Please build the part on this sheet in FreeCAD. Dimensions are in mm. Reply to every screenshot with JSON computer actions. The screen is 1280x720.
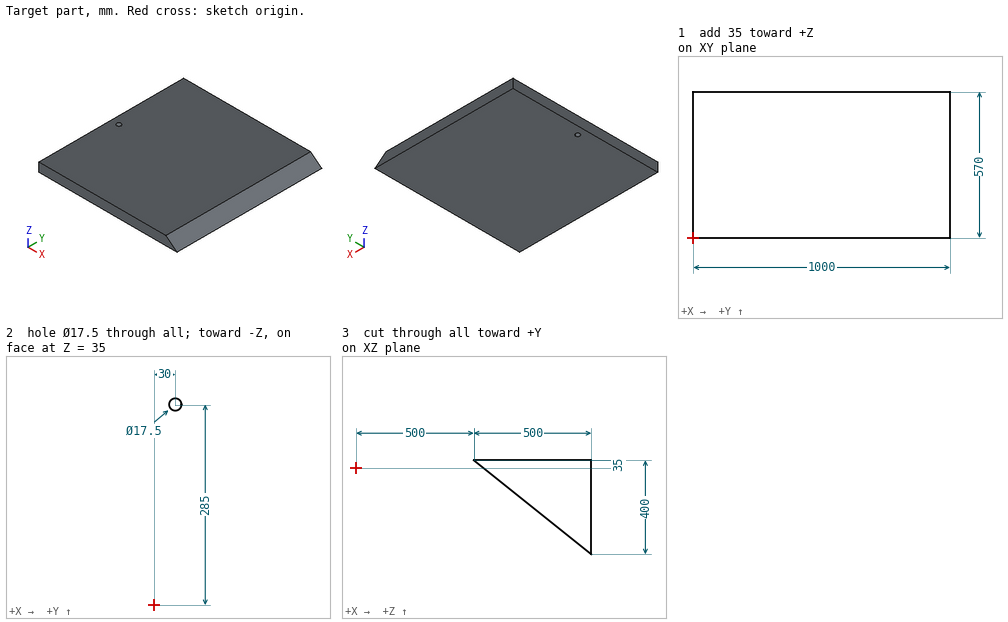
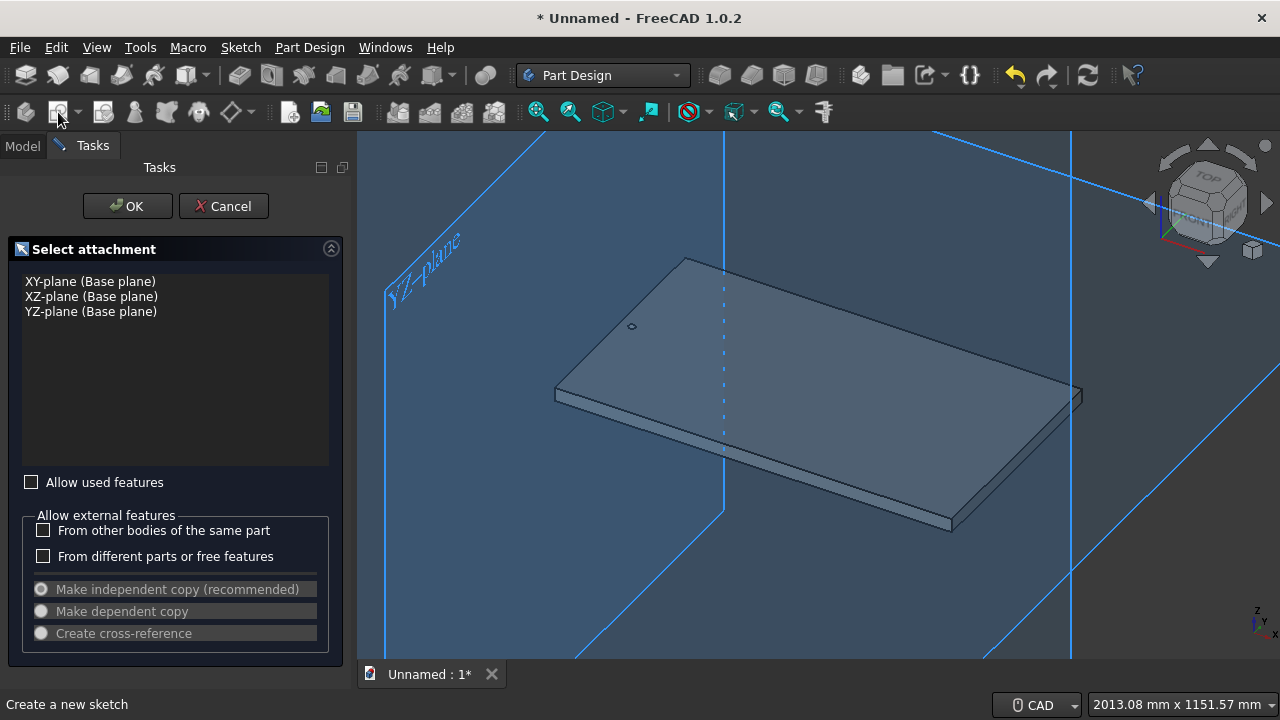
{"action": "left_click", "coordinate": [82, 296]}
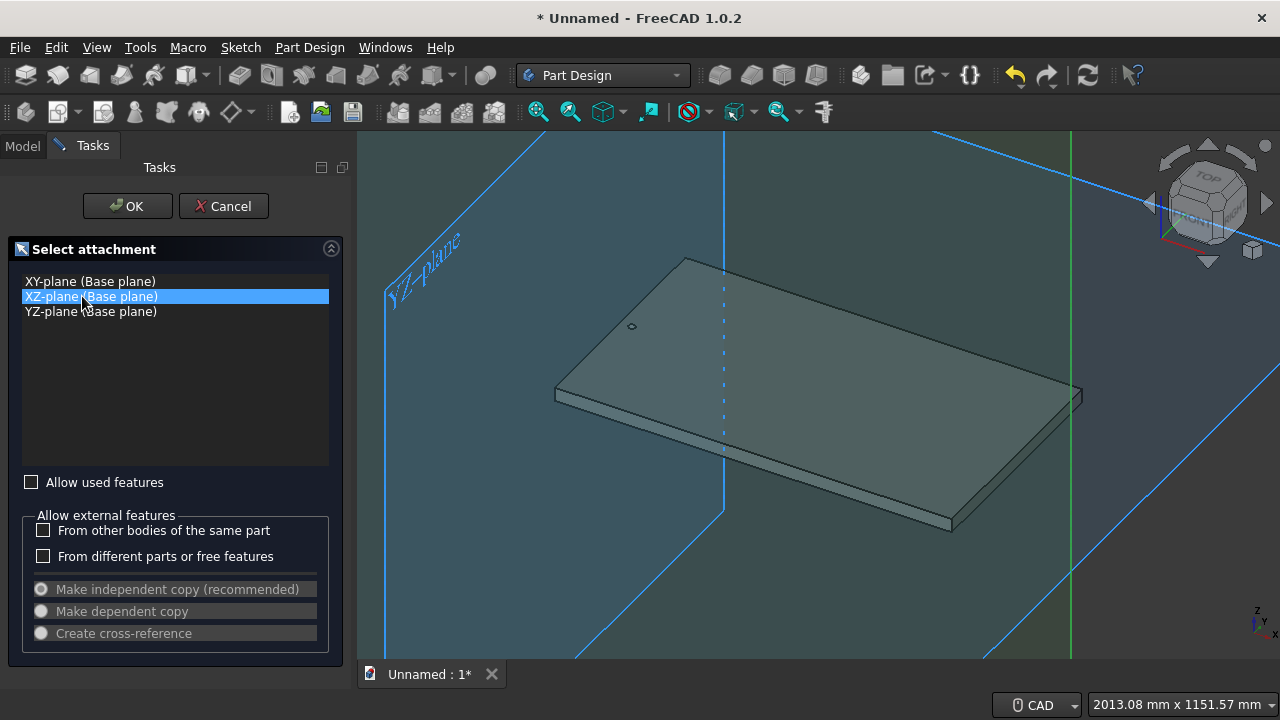
{"action": "left_click", "coordinate": [128, 206]}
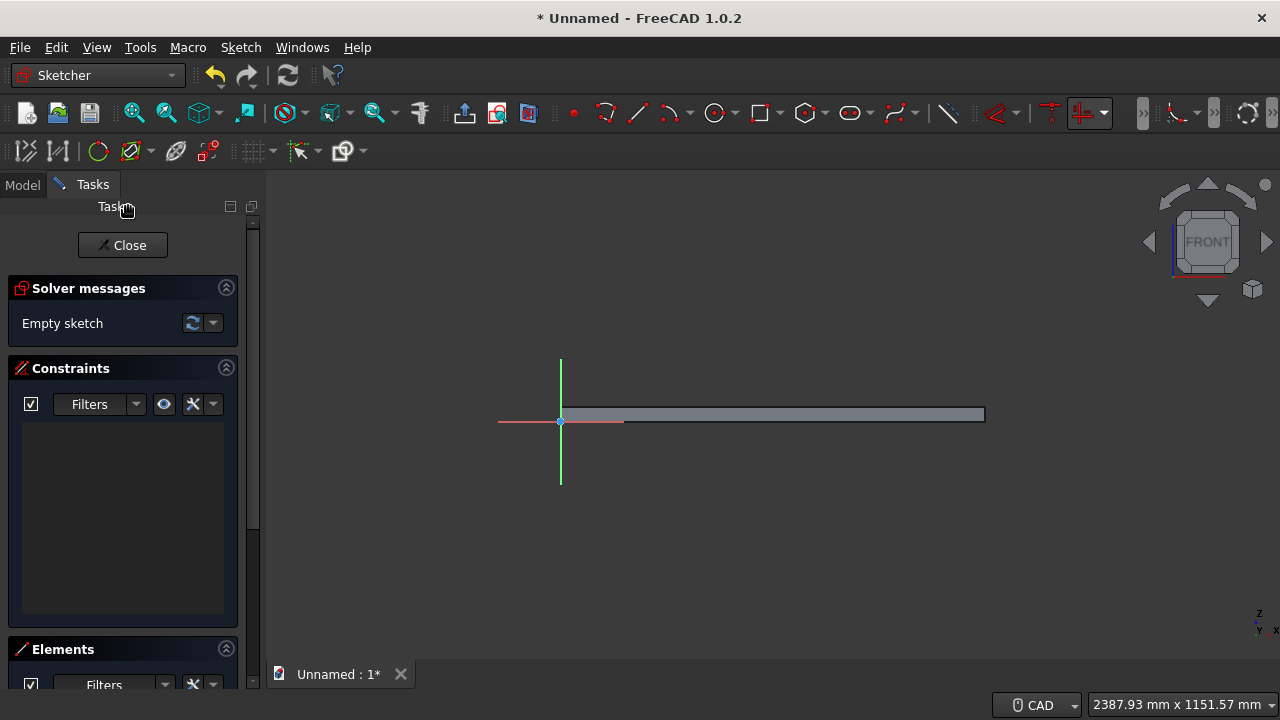
{"action": "scroll", "coordinate": [912, 631], "scroll_direction": "up", "scroll_amount": 2}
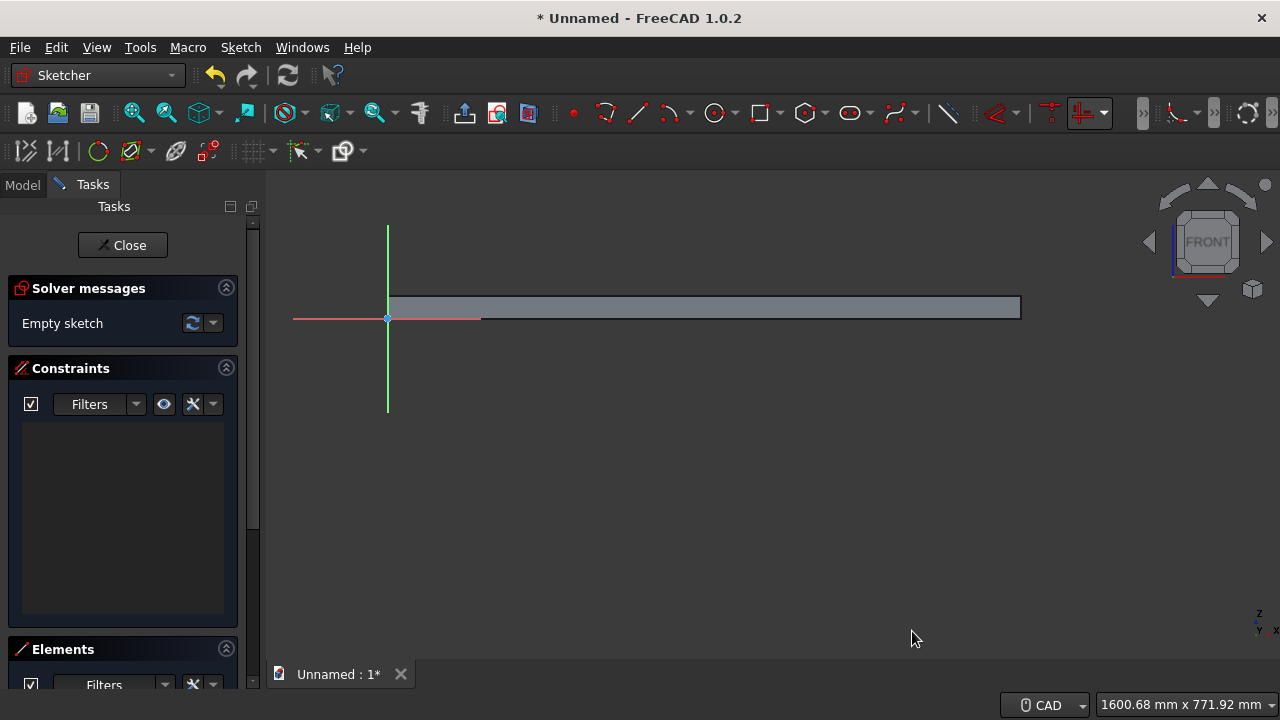
{"action": "left_click", "coordinate": [606, 114]}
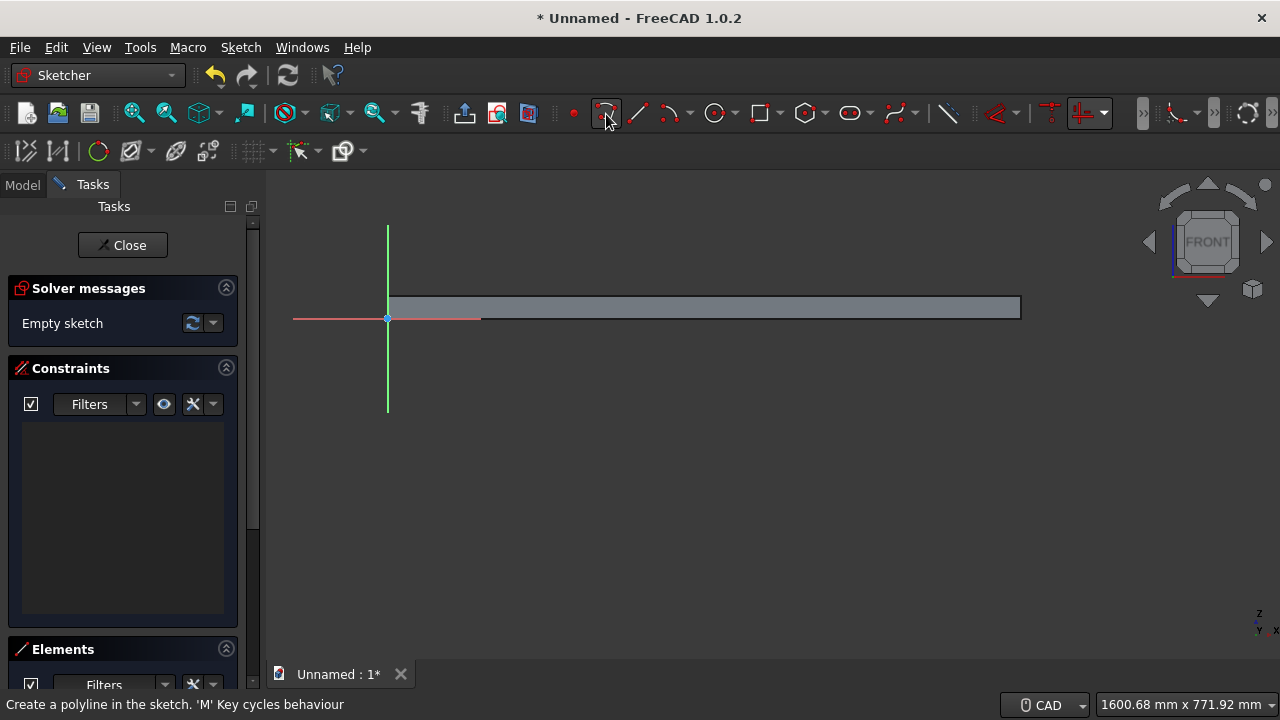
{"action": "left_click", "coordinate": [704, 296]}
{"action": "left_click", "coordinate": [1021, 550]}
{"action": "left_click", "coordinate": [1021, 296]}
{"action": "left_click", "coordinate": [704, 297]}
{"action": "key", "text": "Escape"}
{"action": "key", "text": "Escape"}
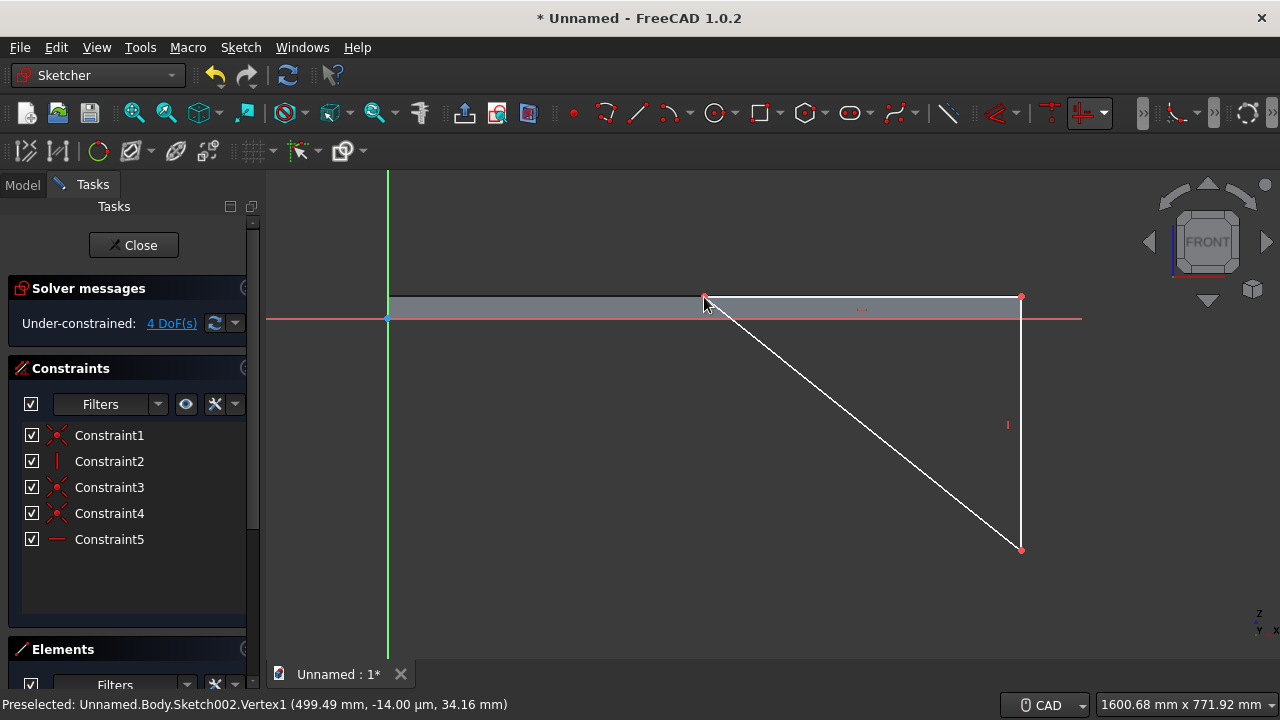
{"action": "key", "text": "d"}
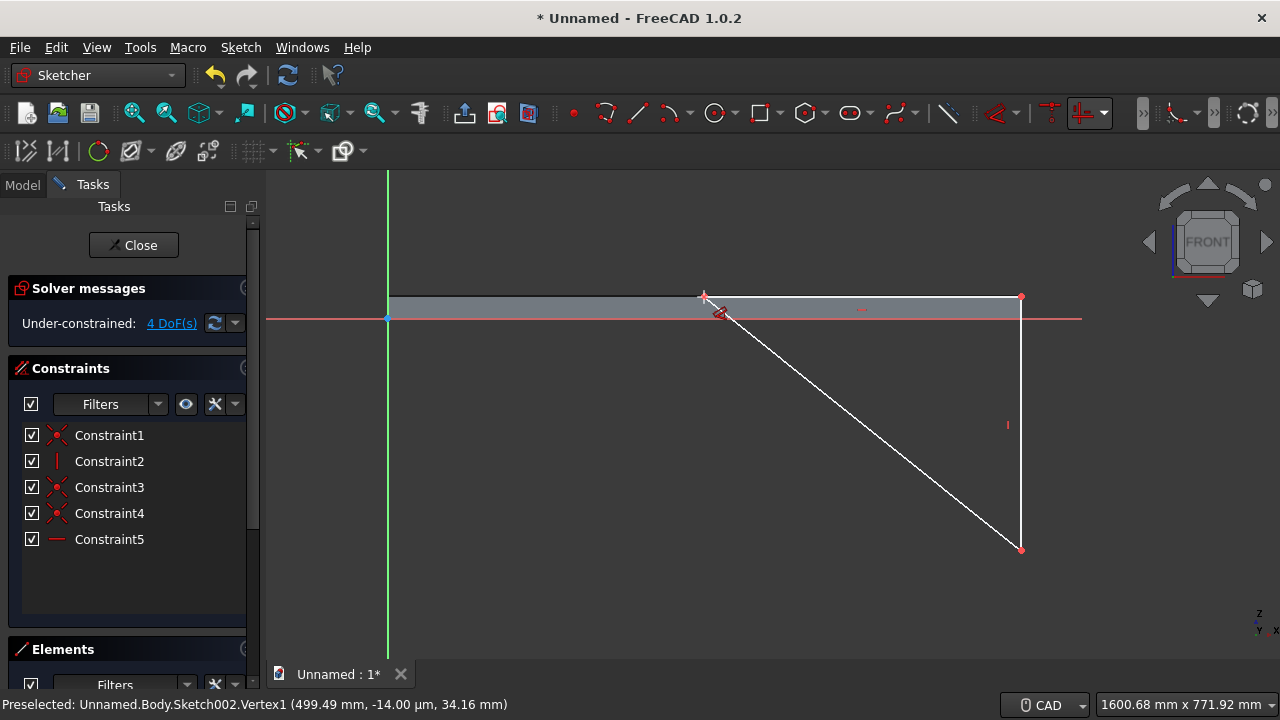
{"action": "left_click", "coordinate": [1021, 475]}
{"action": "left_click", "coordinate": [1055, 424]}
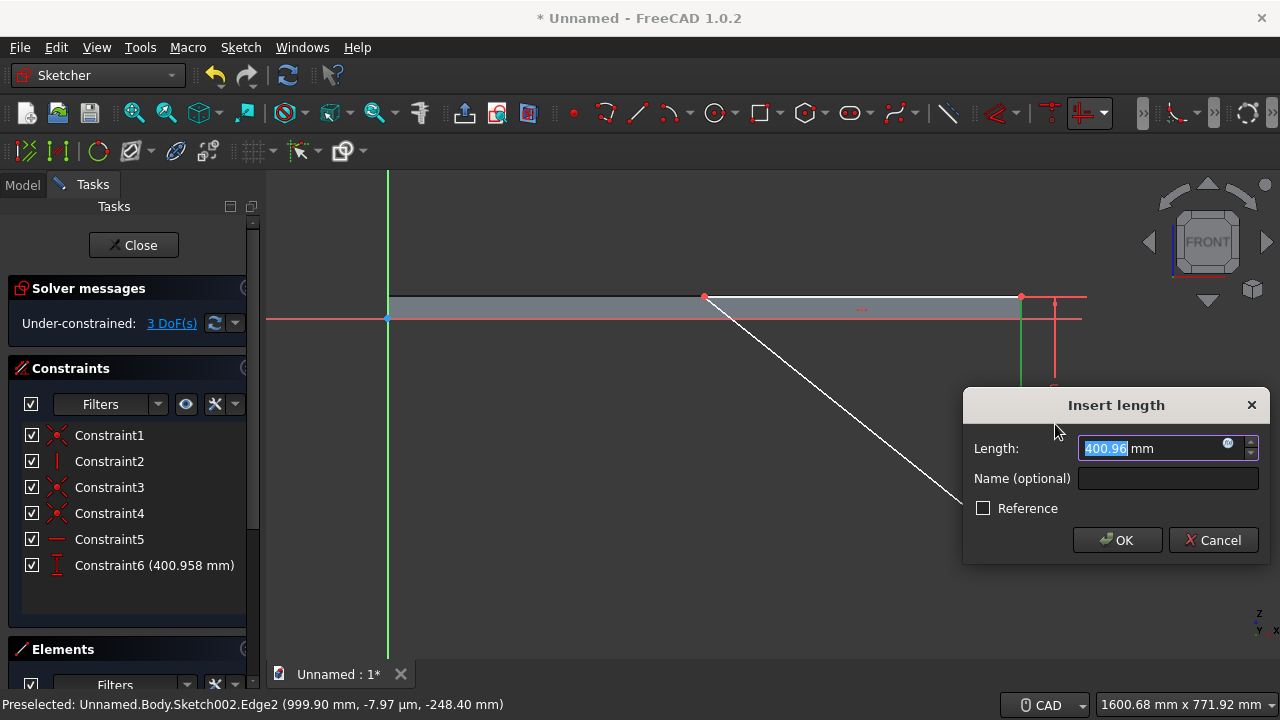
{"action": "type", "text": "400"}
{"action": "key", "text": "Return"}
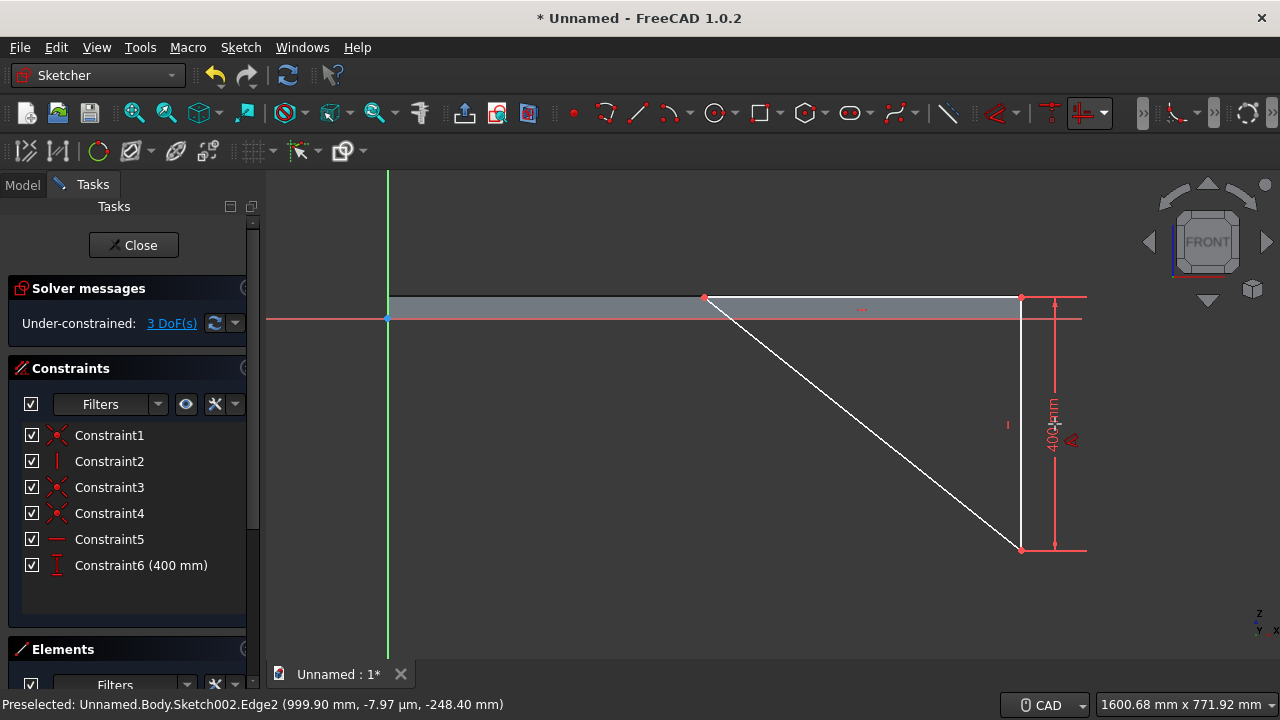
{"action": "left_click", "coordinate": [926, 297]}
{"action": "left_click", "coordinate": [862, 263]}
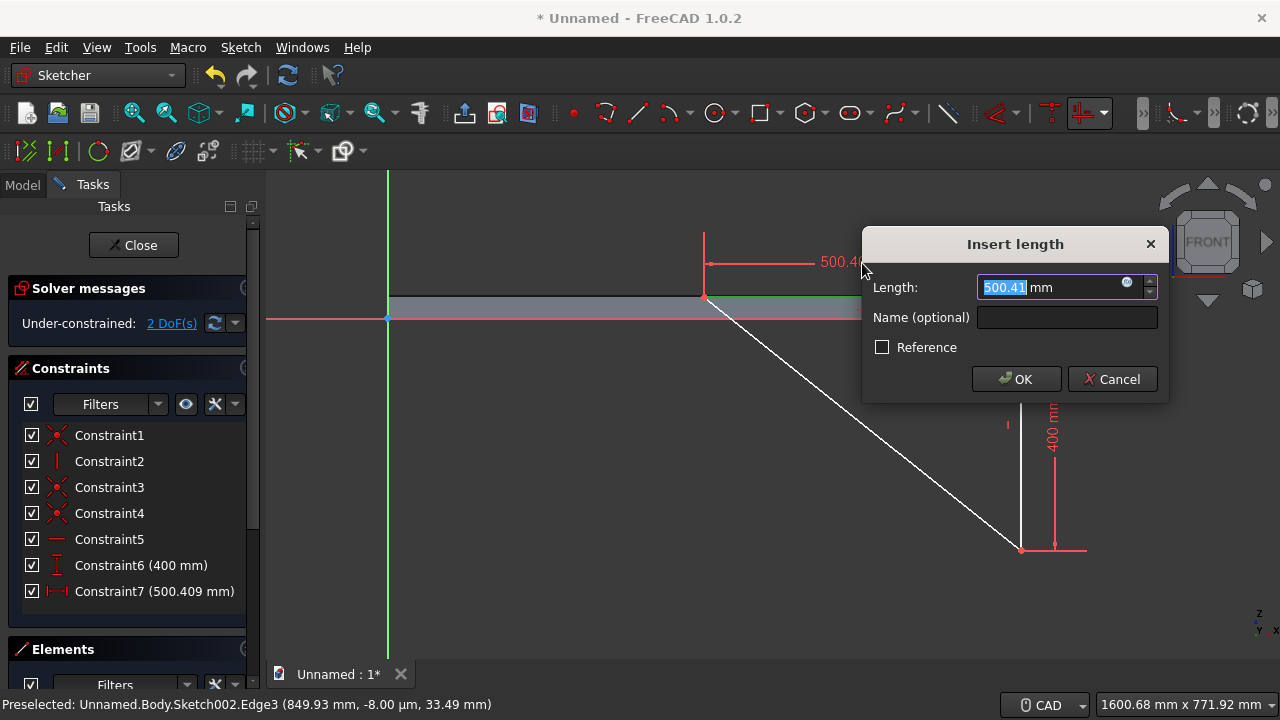
{"action": "type", "text": "500"}
{"action": "key", "text": "Return"}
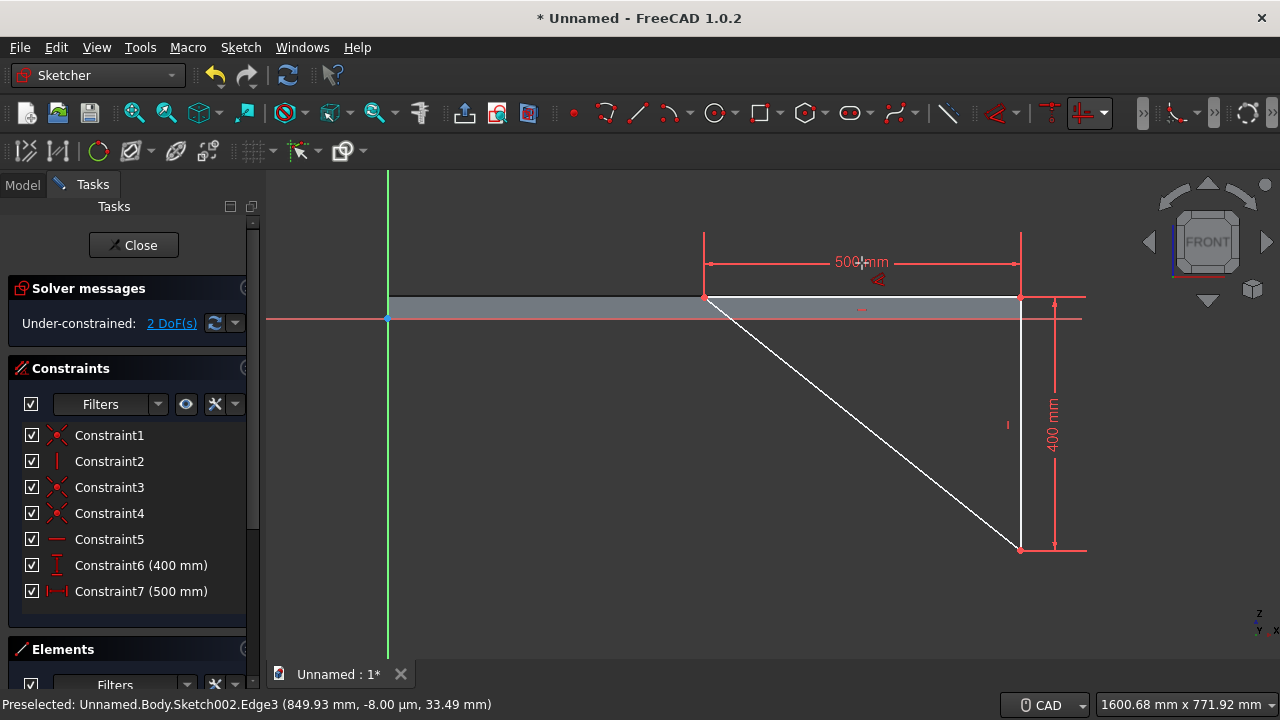
{"action": "scroll", "coordinate": [704, 297], "scroll_direction": "up", "scroll_amount": 3}